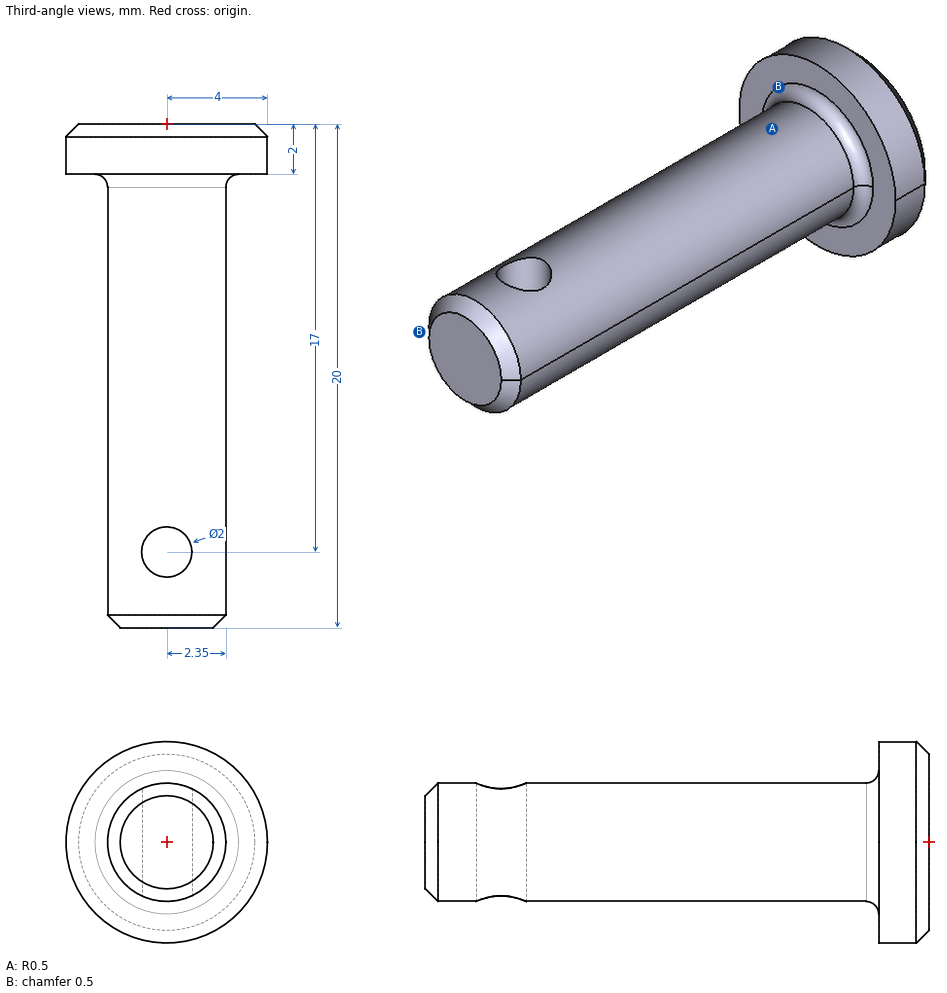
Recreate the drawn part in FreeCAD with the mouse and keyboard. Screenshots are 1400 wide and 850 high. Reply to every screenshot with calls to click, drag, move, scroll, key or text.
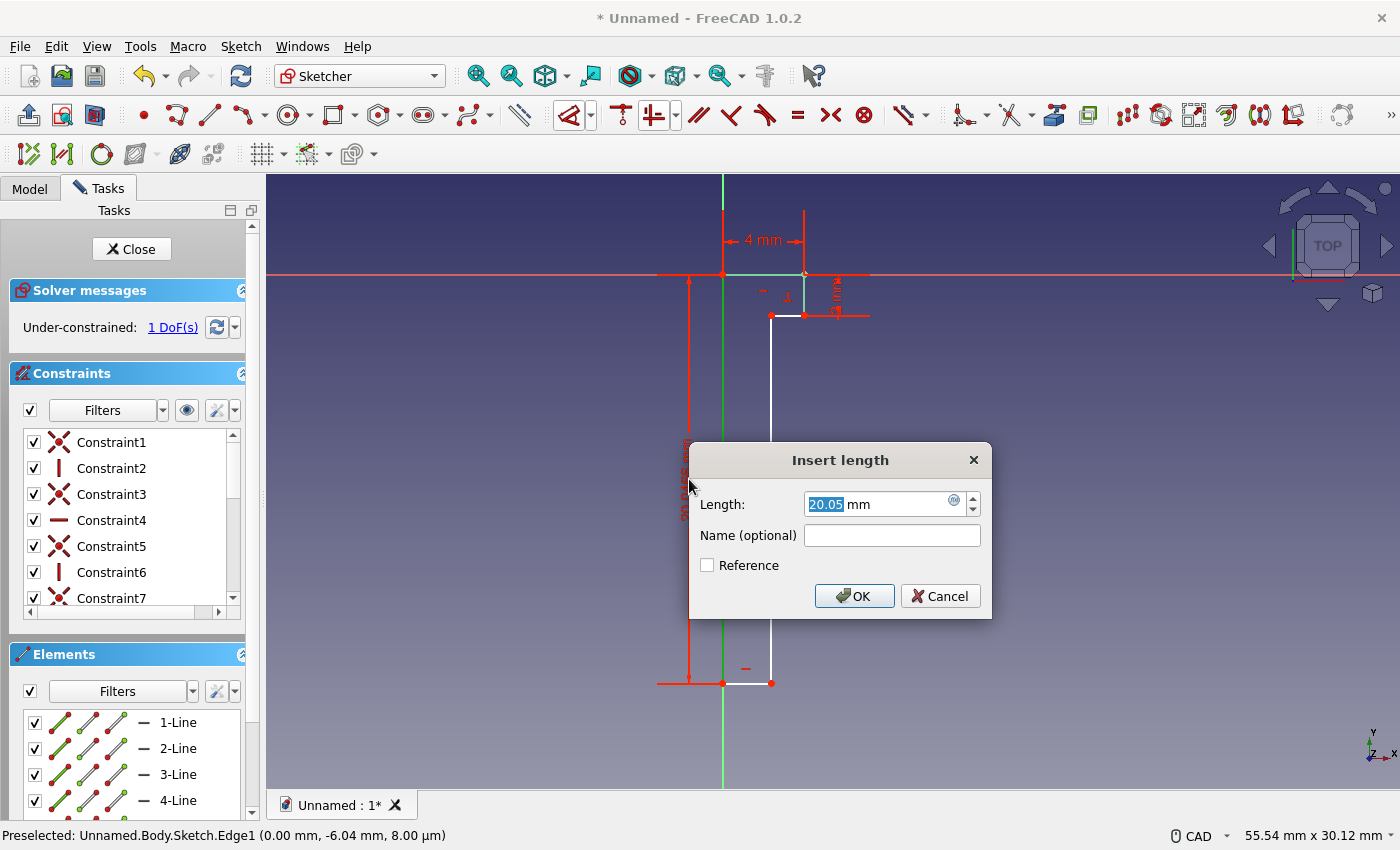
text(20)
key(Return)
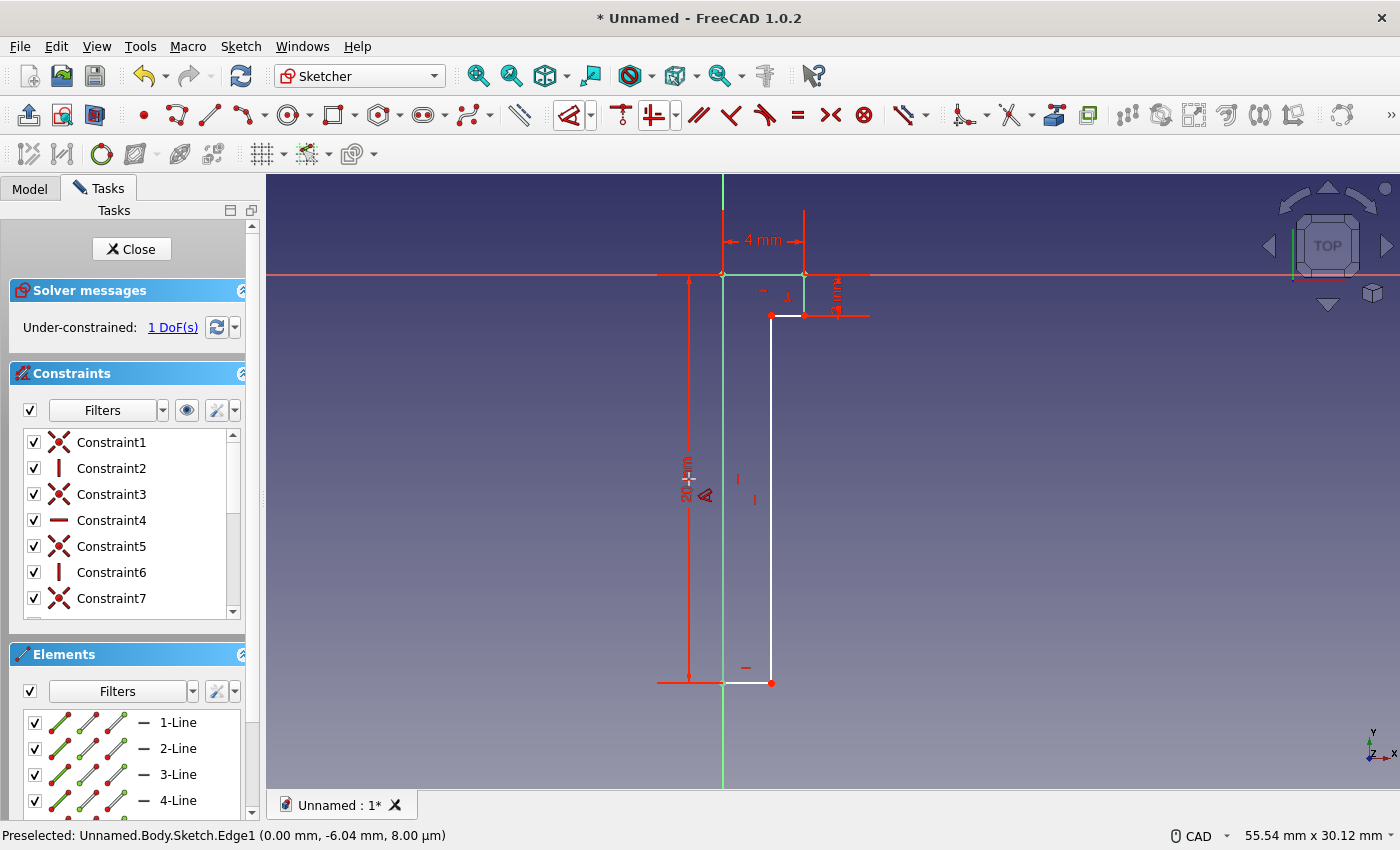
click(737, 683)
click(747, 717)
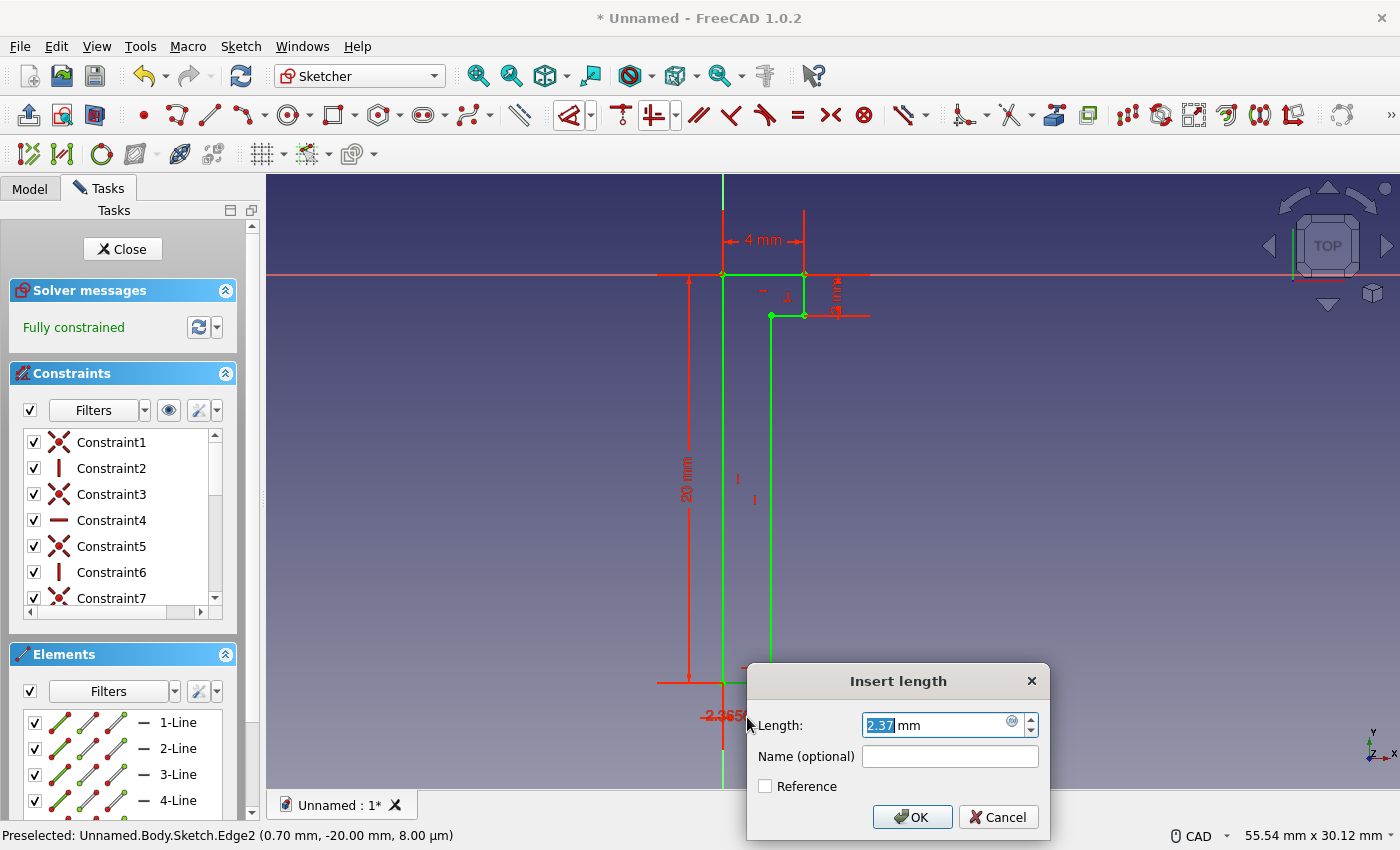
text(2.35)
key(Return)
key(Escape)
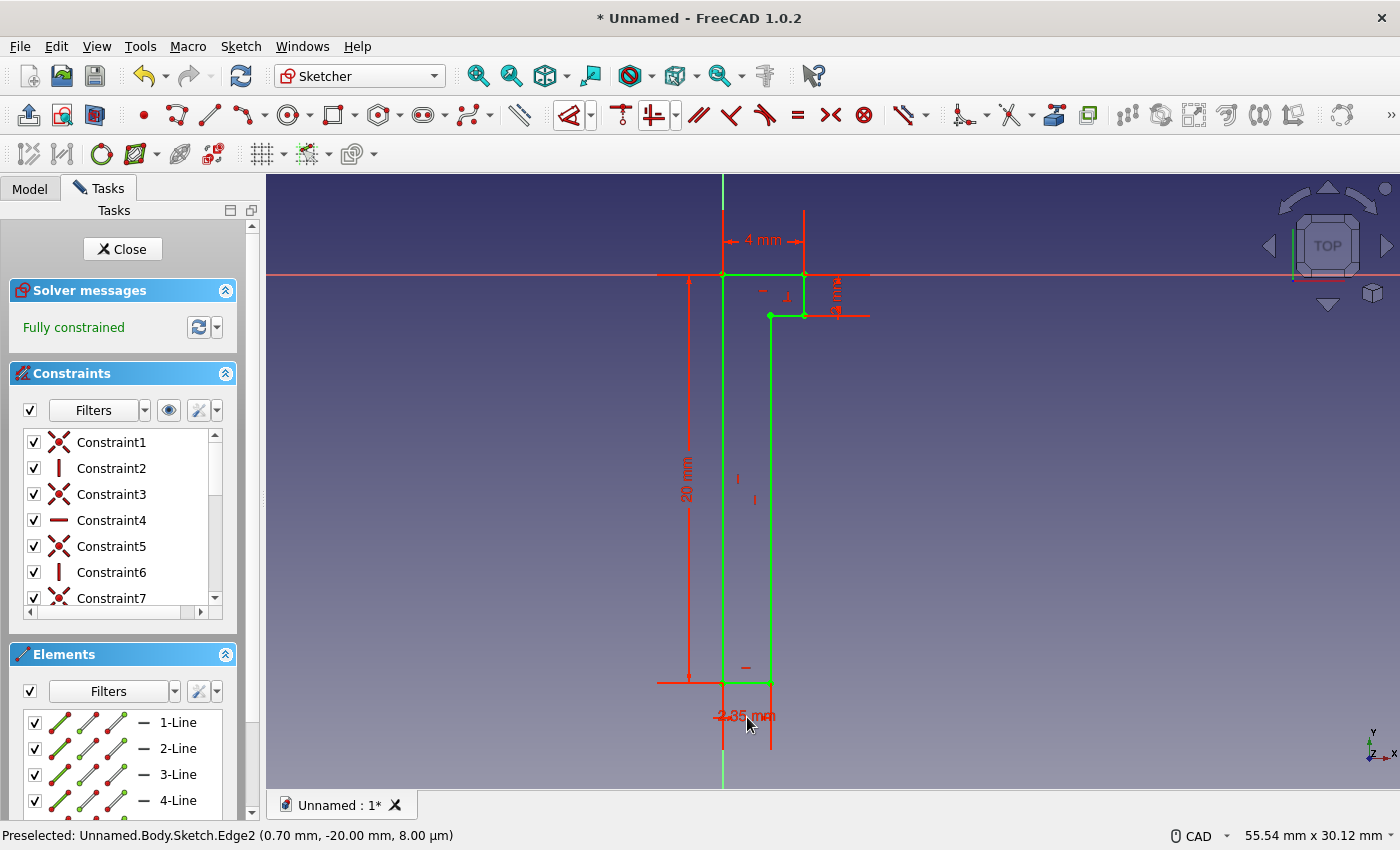
click(123, 249)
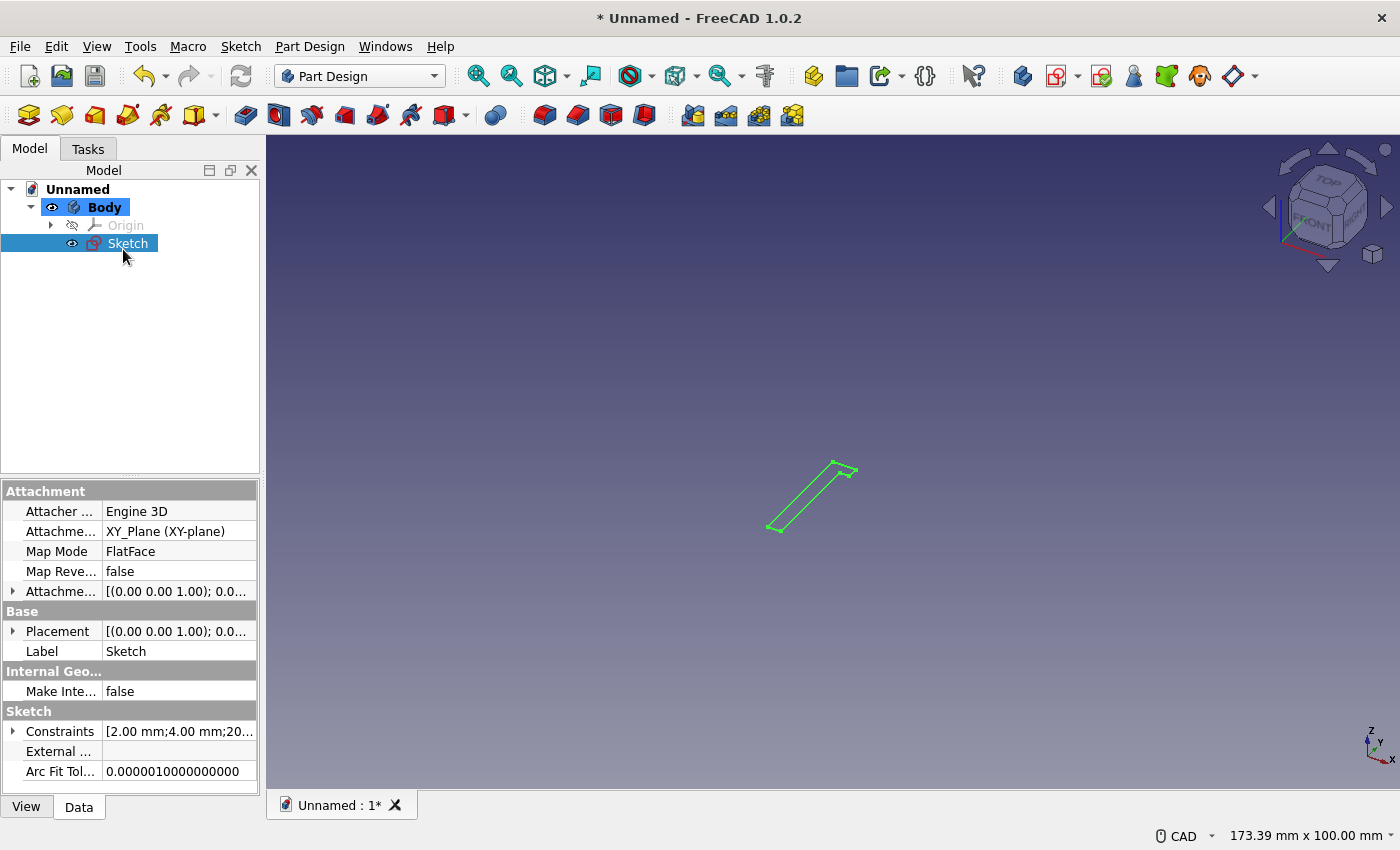
click(62, 116)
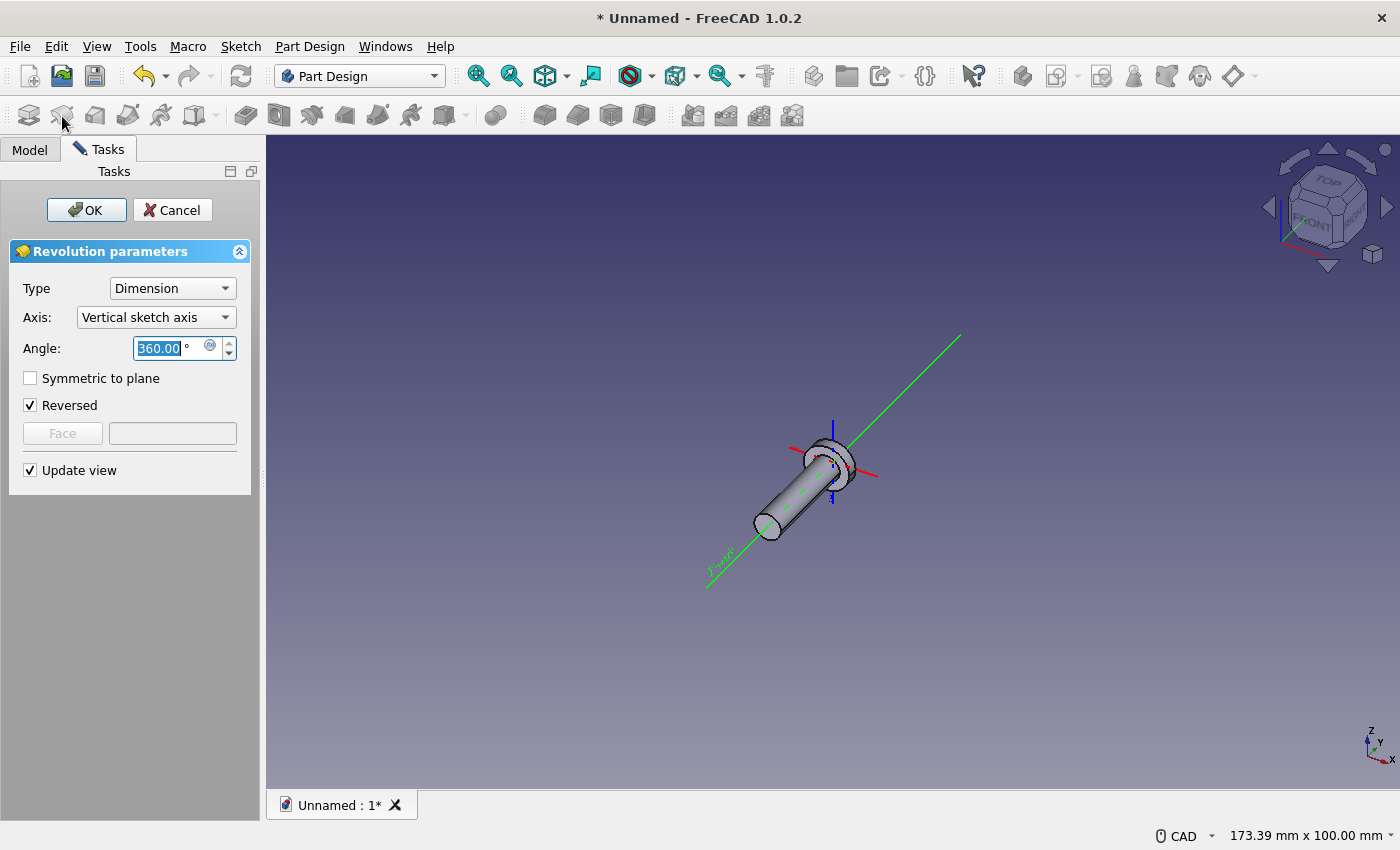
click(87, 210)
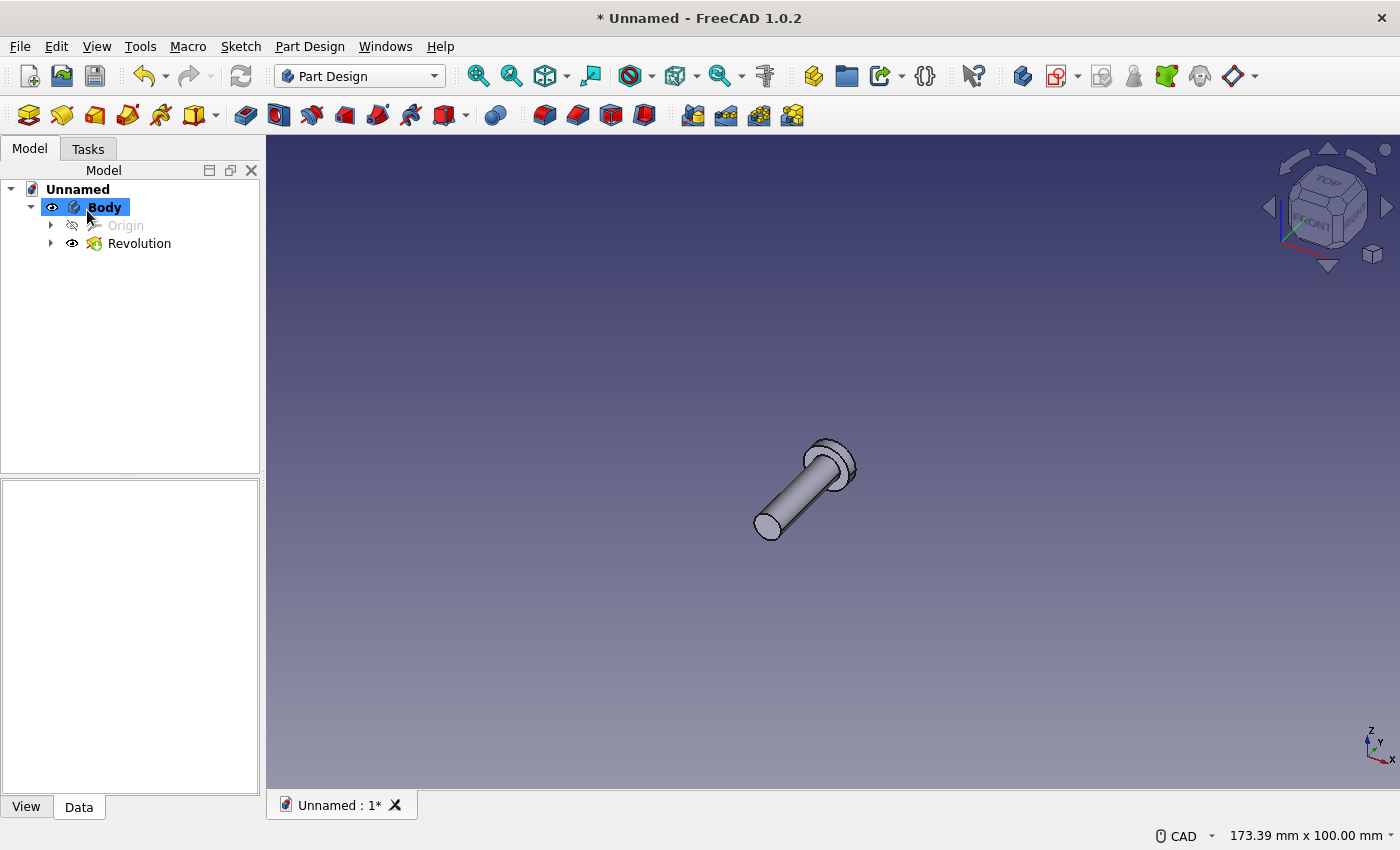
key(v)
key(f)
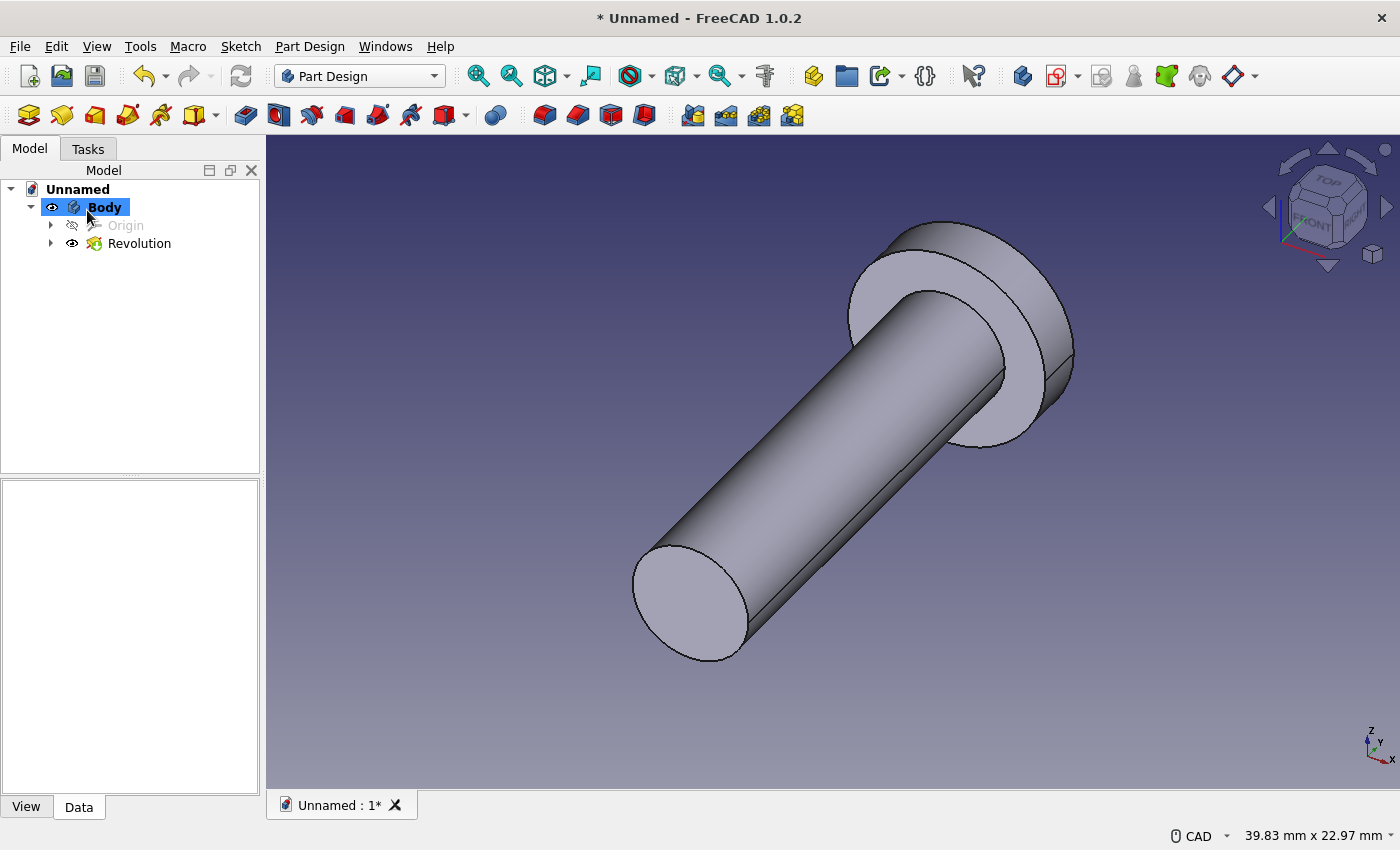
key(0)